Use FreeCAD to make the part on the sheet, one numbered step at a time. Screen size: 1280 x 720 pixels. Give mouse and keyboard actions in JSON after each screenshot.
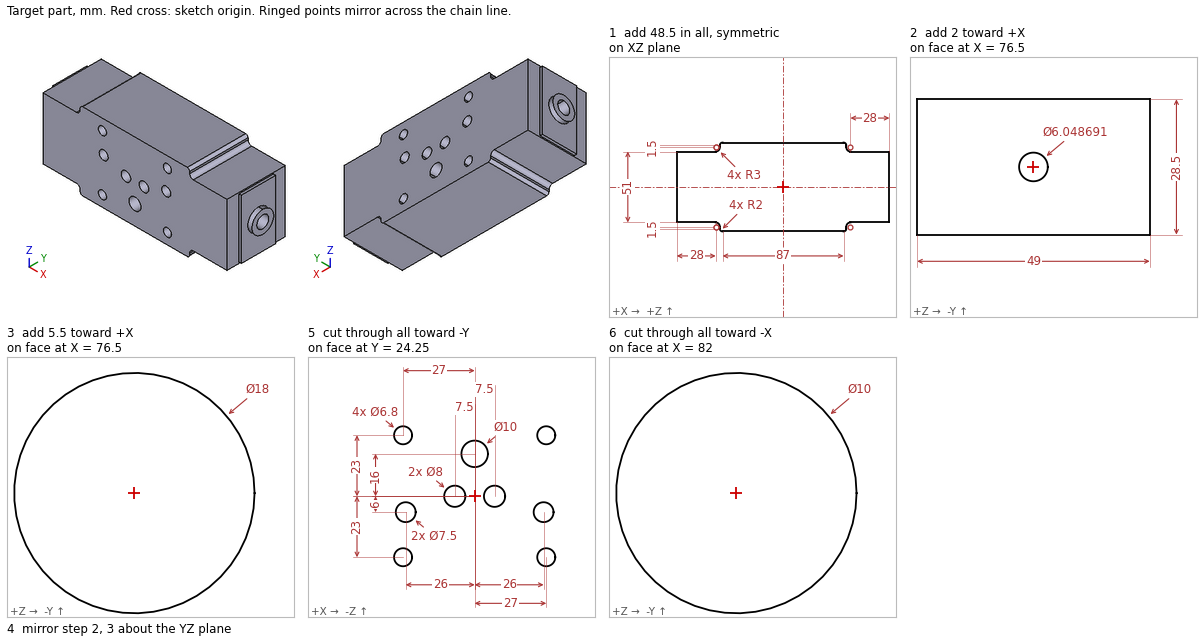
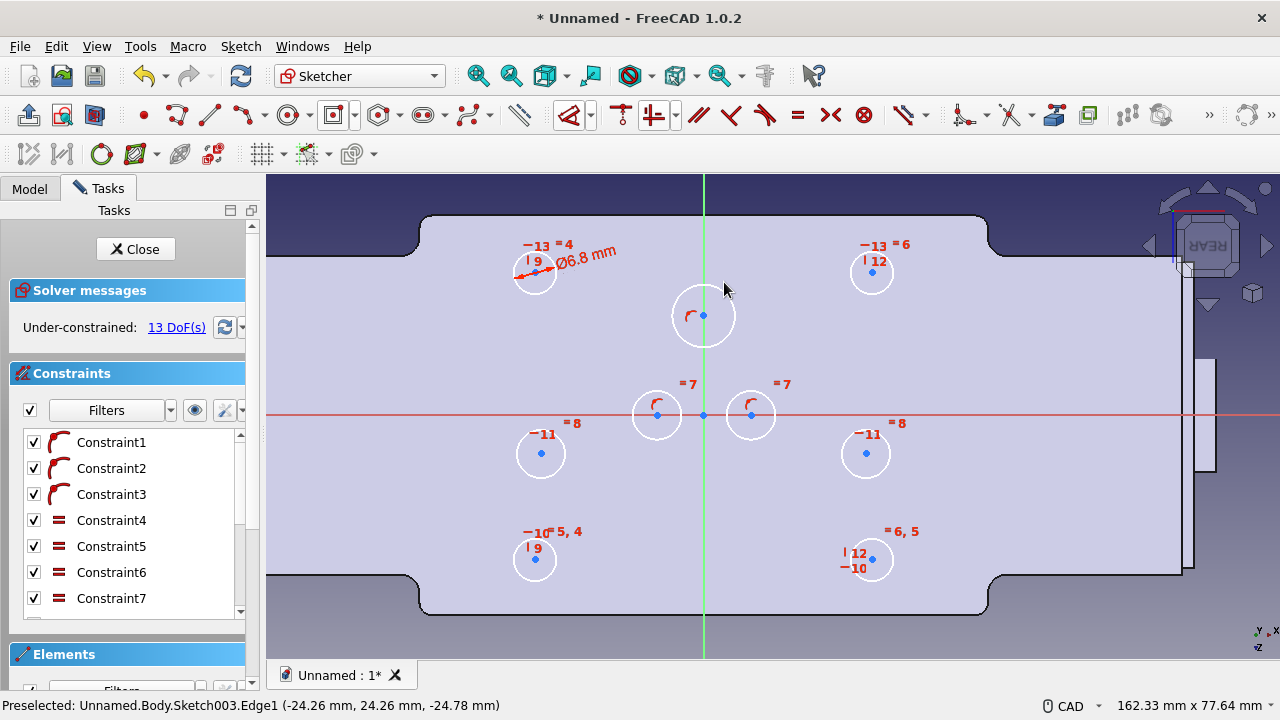
{"action": "left_click", "coordinate": [726, 294]}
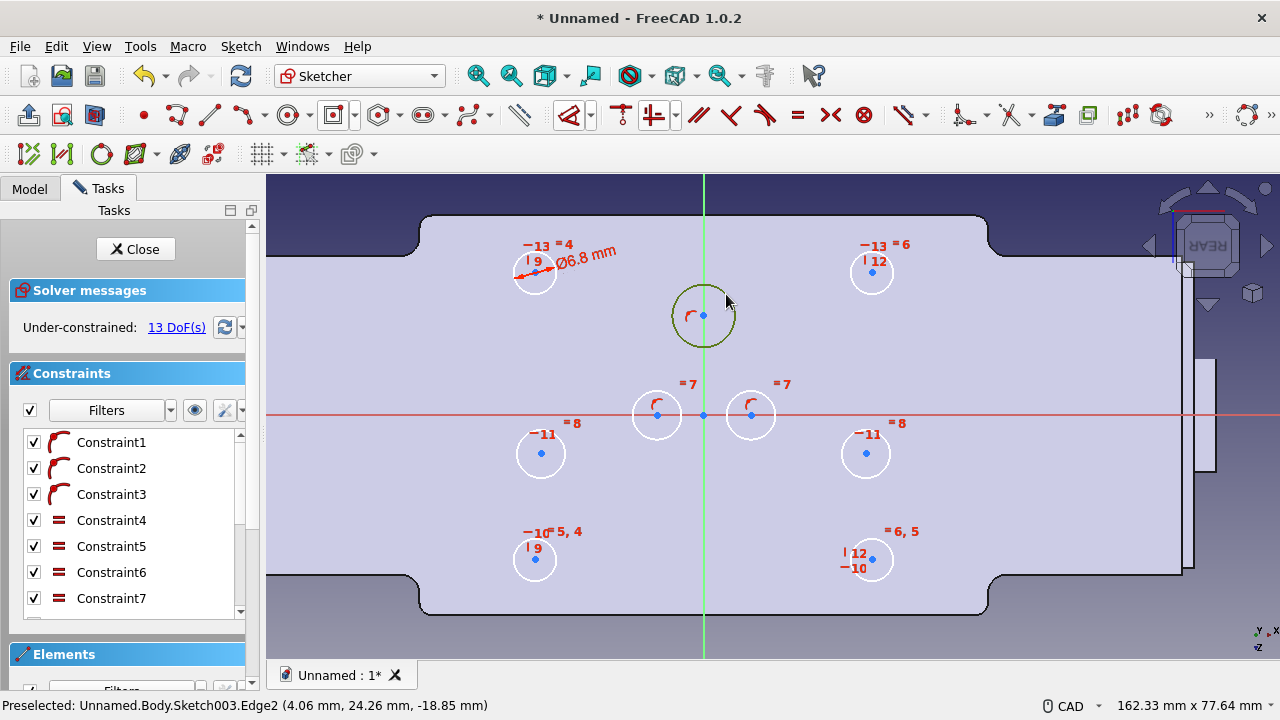
{"action": "key", "text": "k o"}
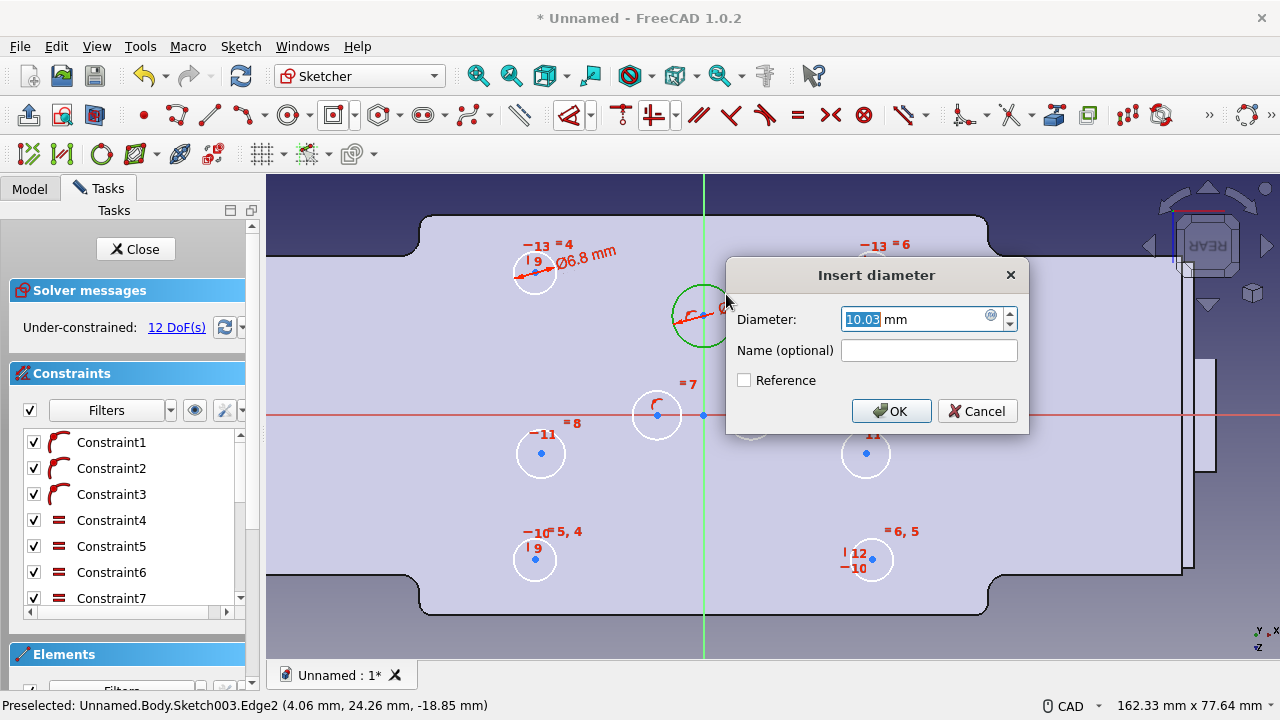
{"action": "type", "text": "10"}
{"action": "key", "text": "Return"}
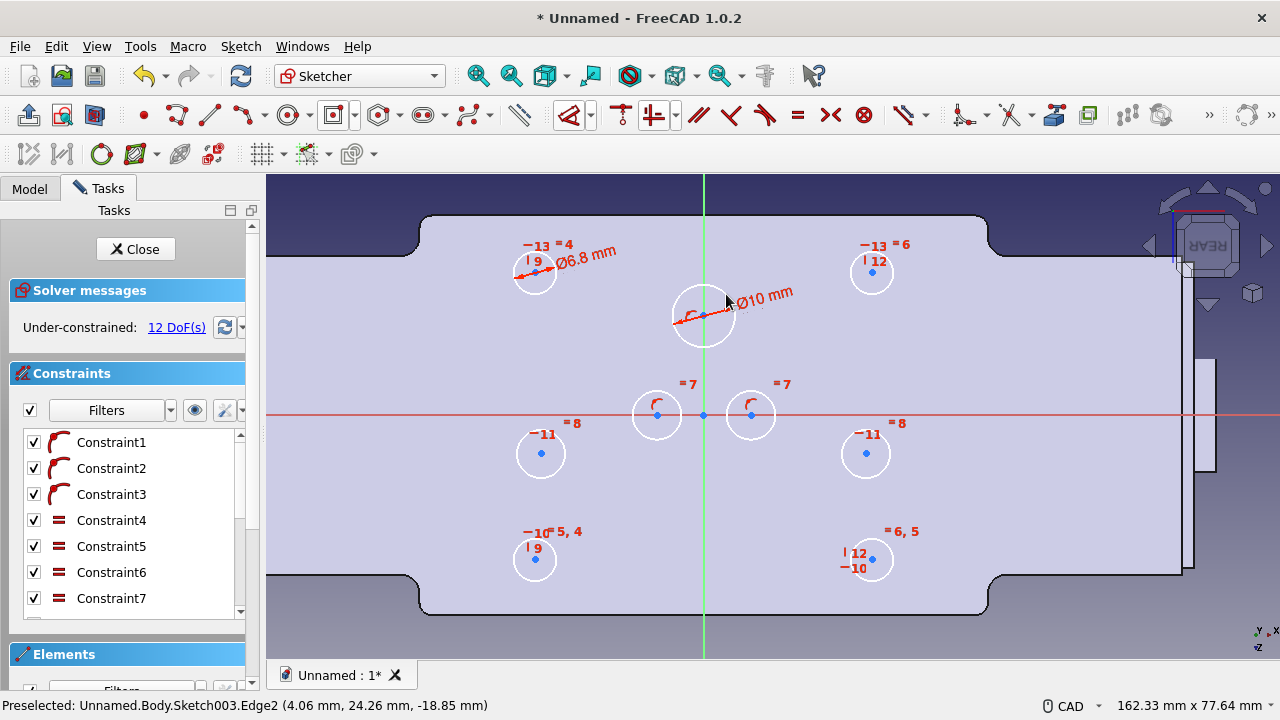
{"action": "left_click", "coordinate": [674, 398]}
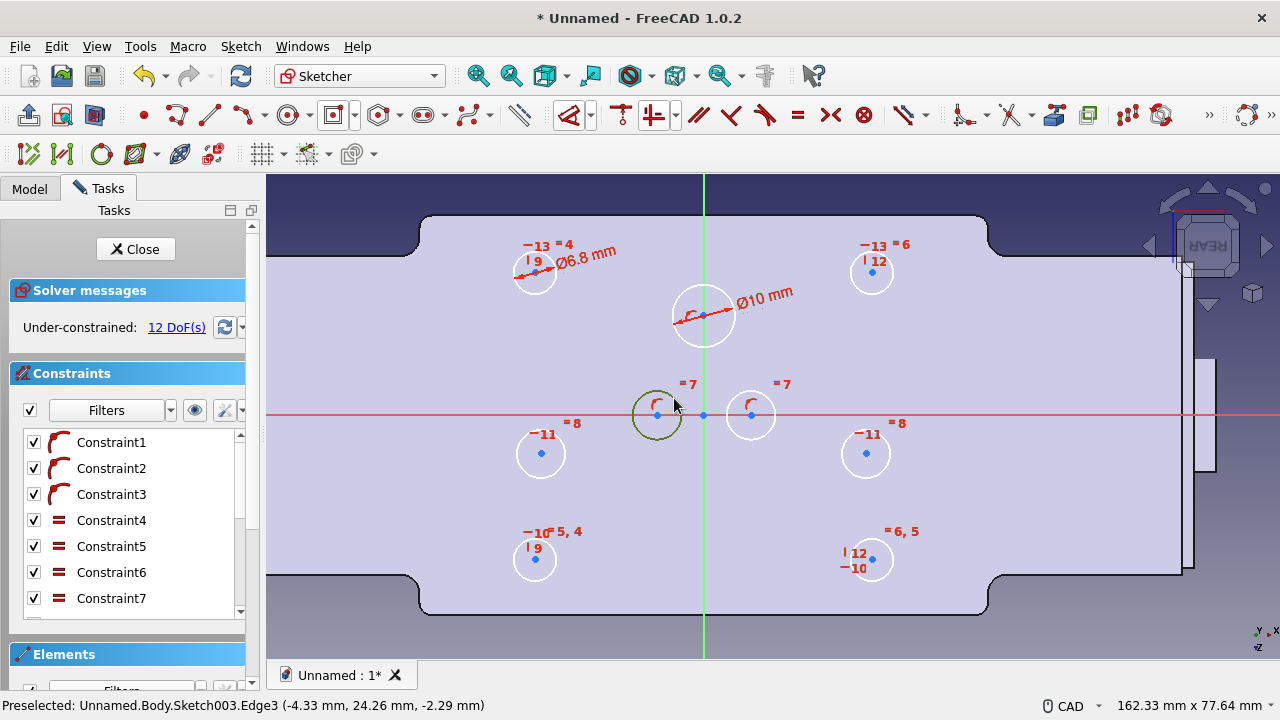
{"action": "key", "text": "k o"}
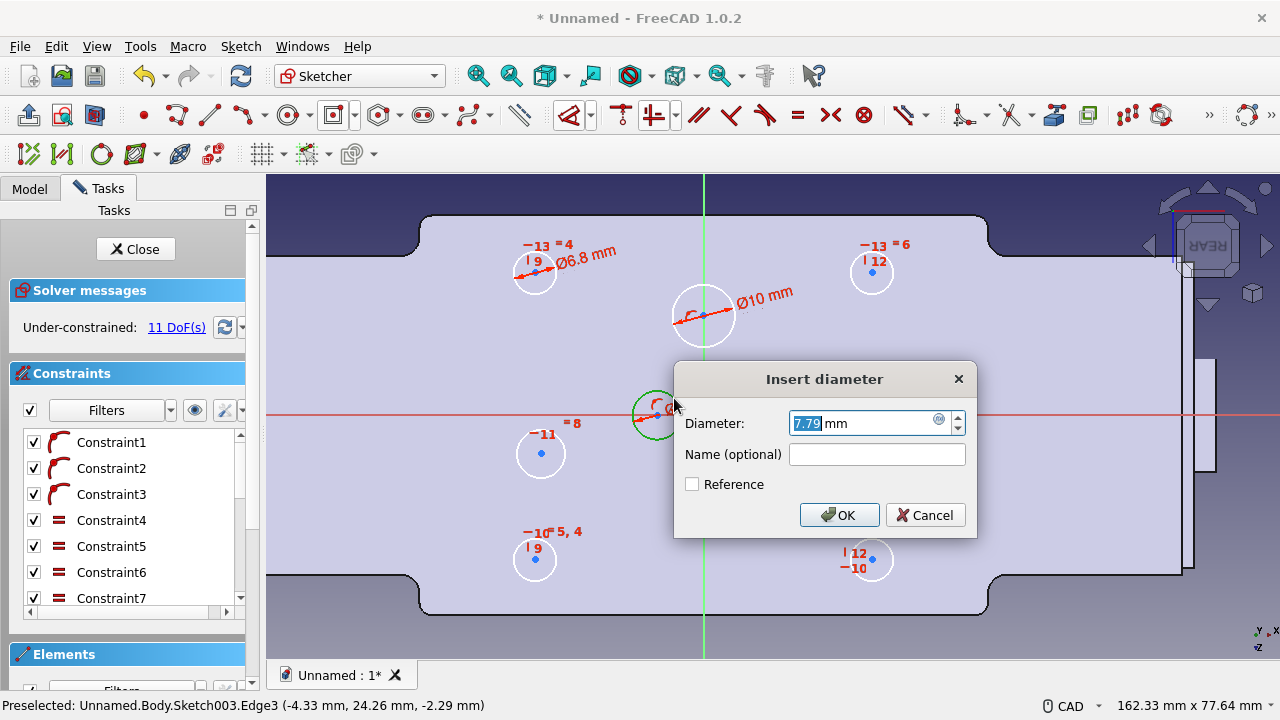
{"action": "type", "text": "8"}
{"action": "key", "text": "Return"}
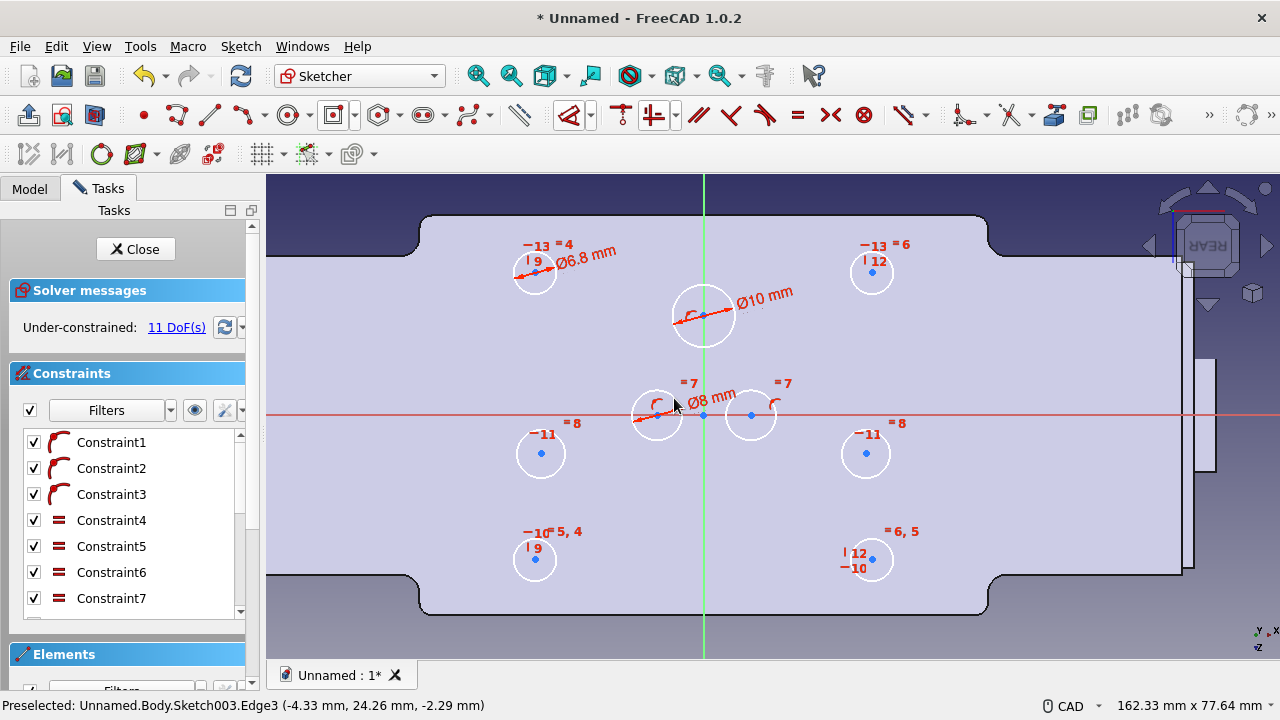
{"action": "left_click", "coordinate": [558, 437]}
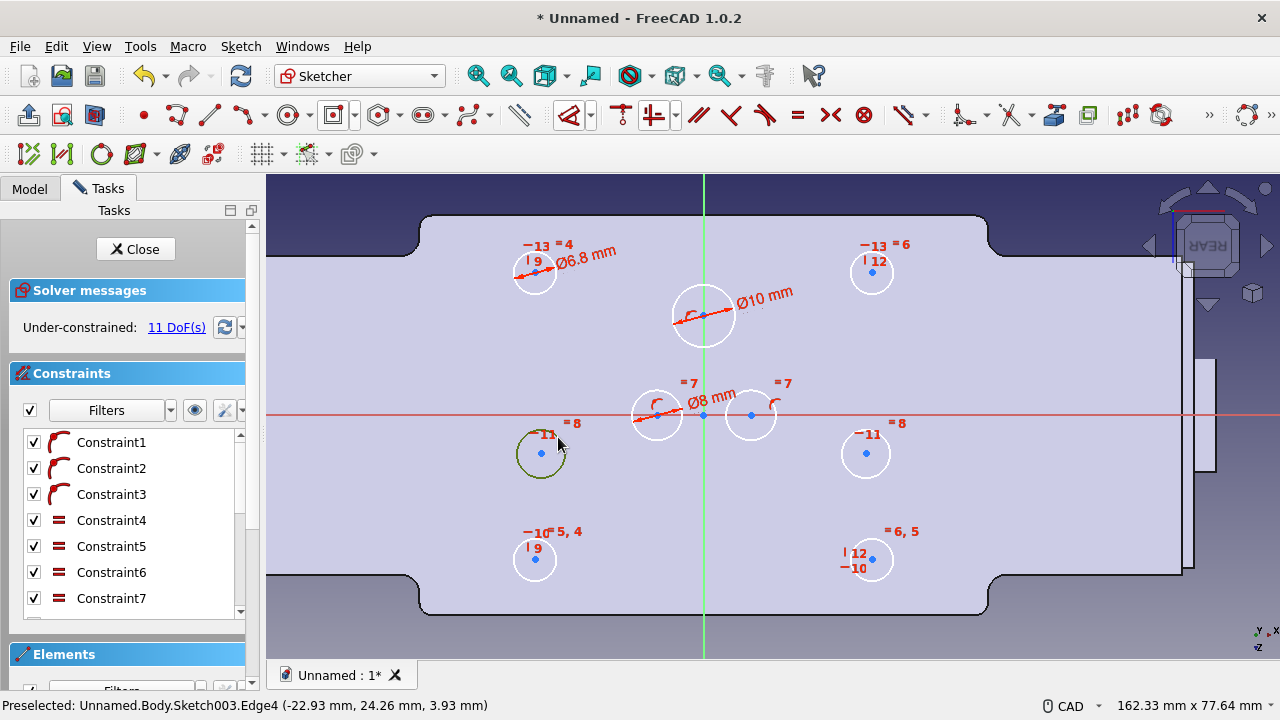
{"action": "key", "text": "k o"}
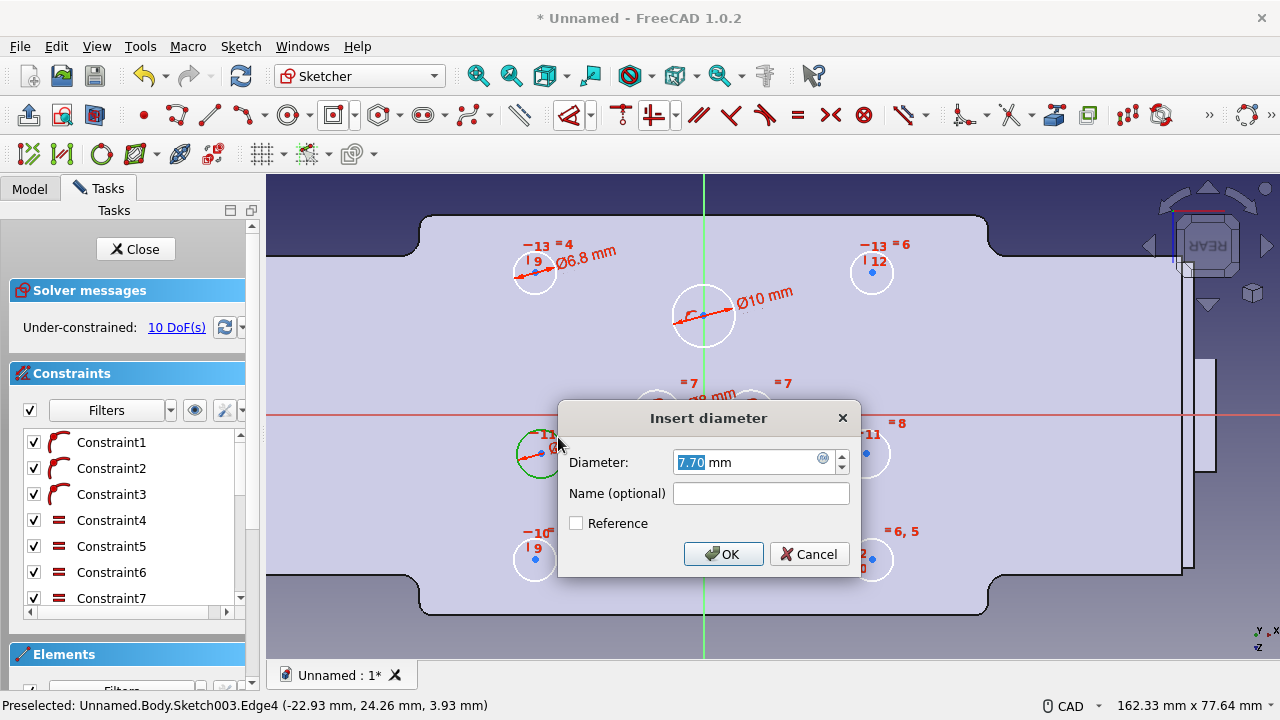
{"action": "type", "text": "7.5"}
{"action": "key", "text": "Return"}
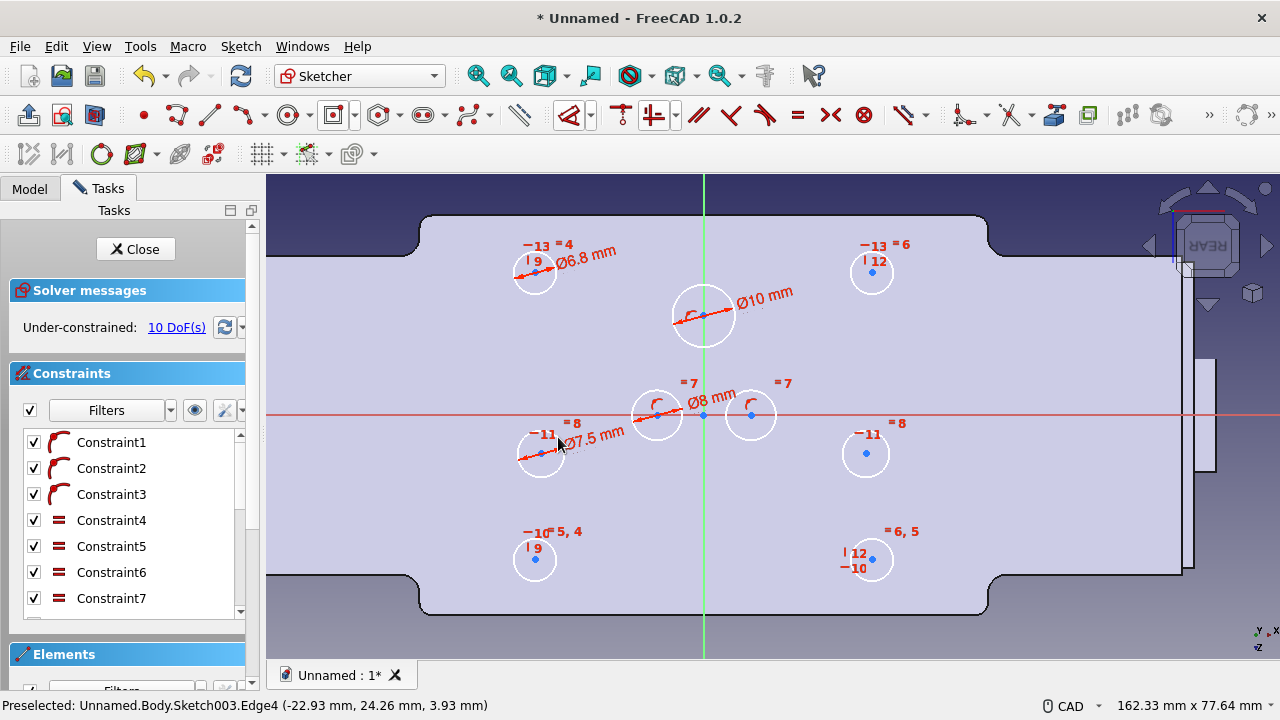
{"action": "left_click", "coordinate": [541, 454]}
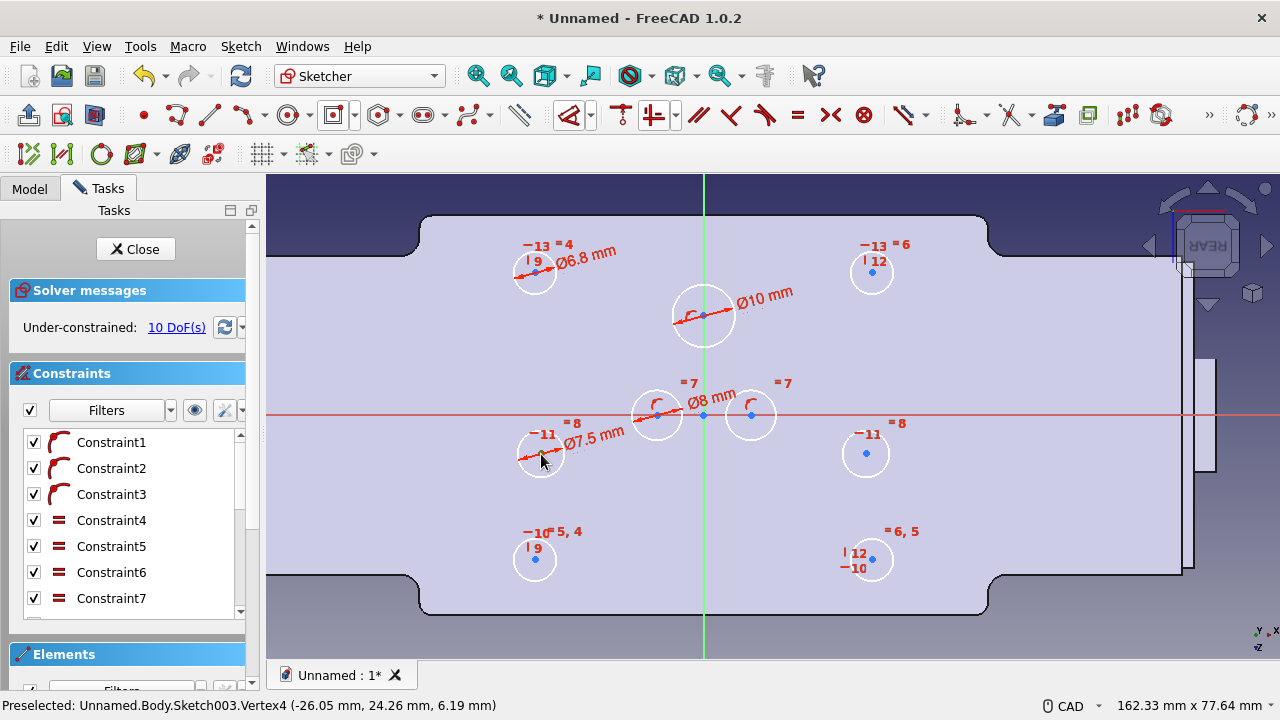
{"action": "key", "text": "i"}